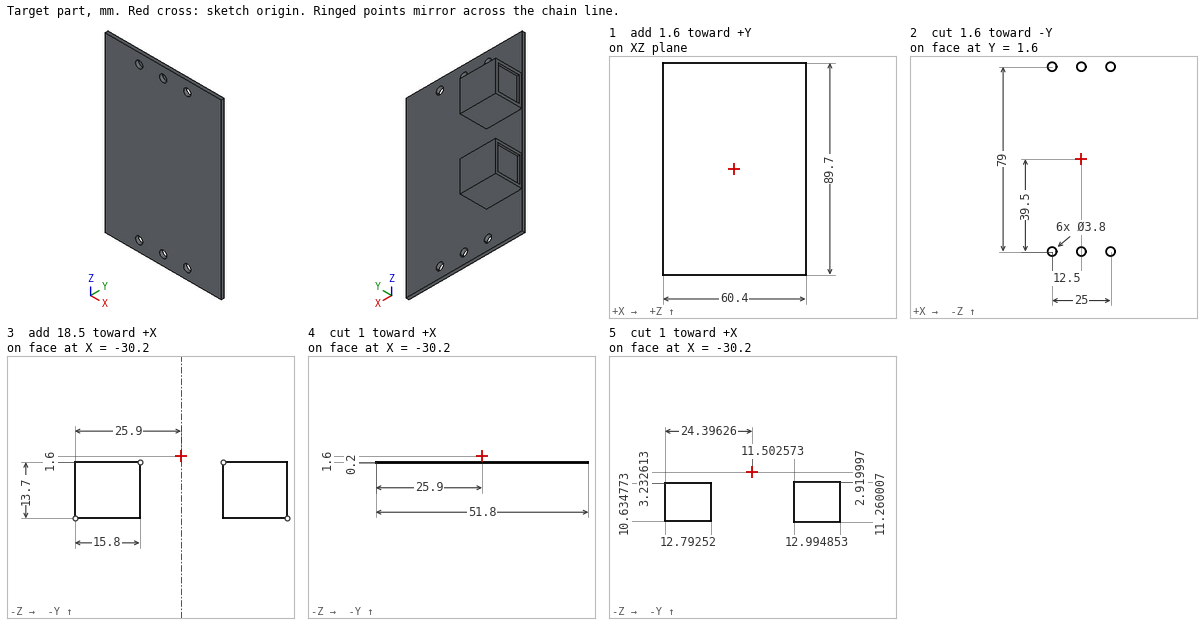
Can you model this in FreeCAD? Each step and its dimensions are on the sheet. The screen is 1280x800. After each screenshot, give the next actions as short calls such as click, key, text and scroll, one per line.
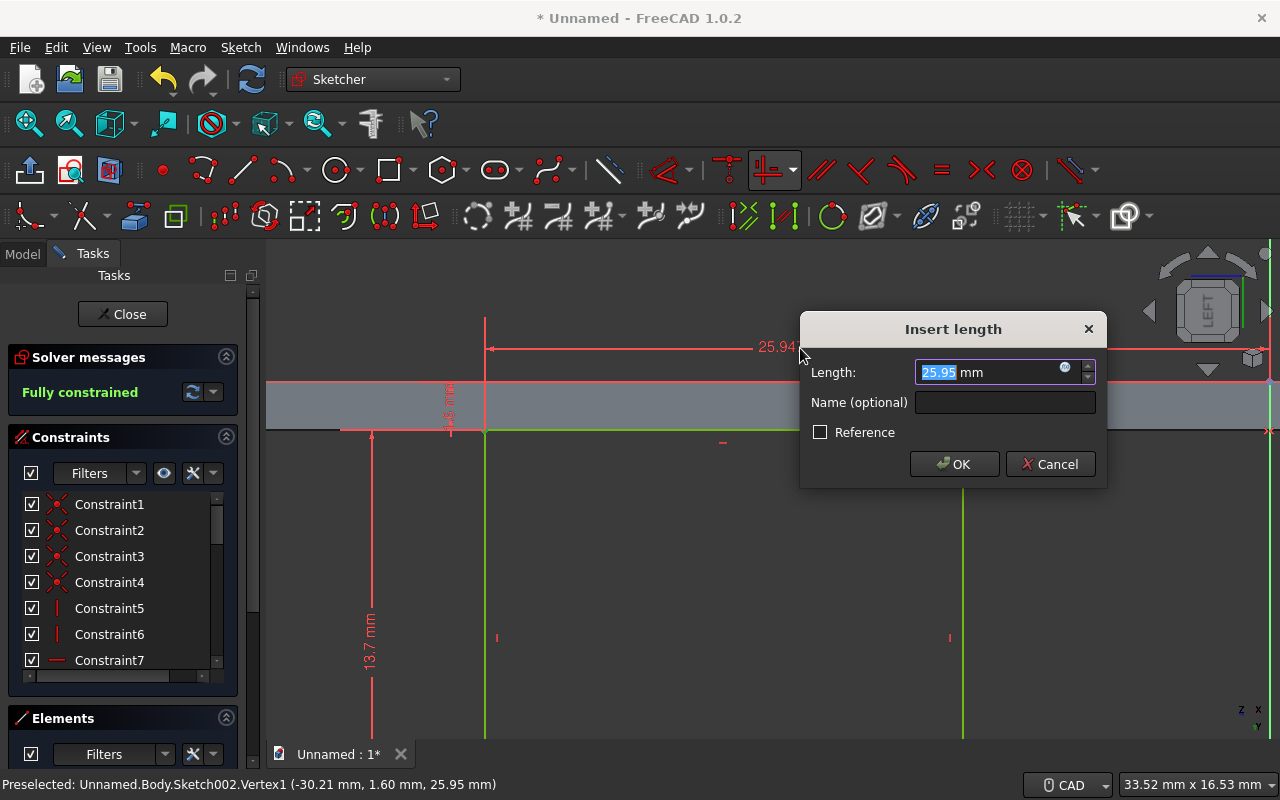
text(25.9)
key(Return)
key(Escape)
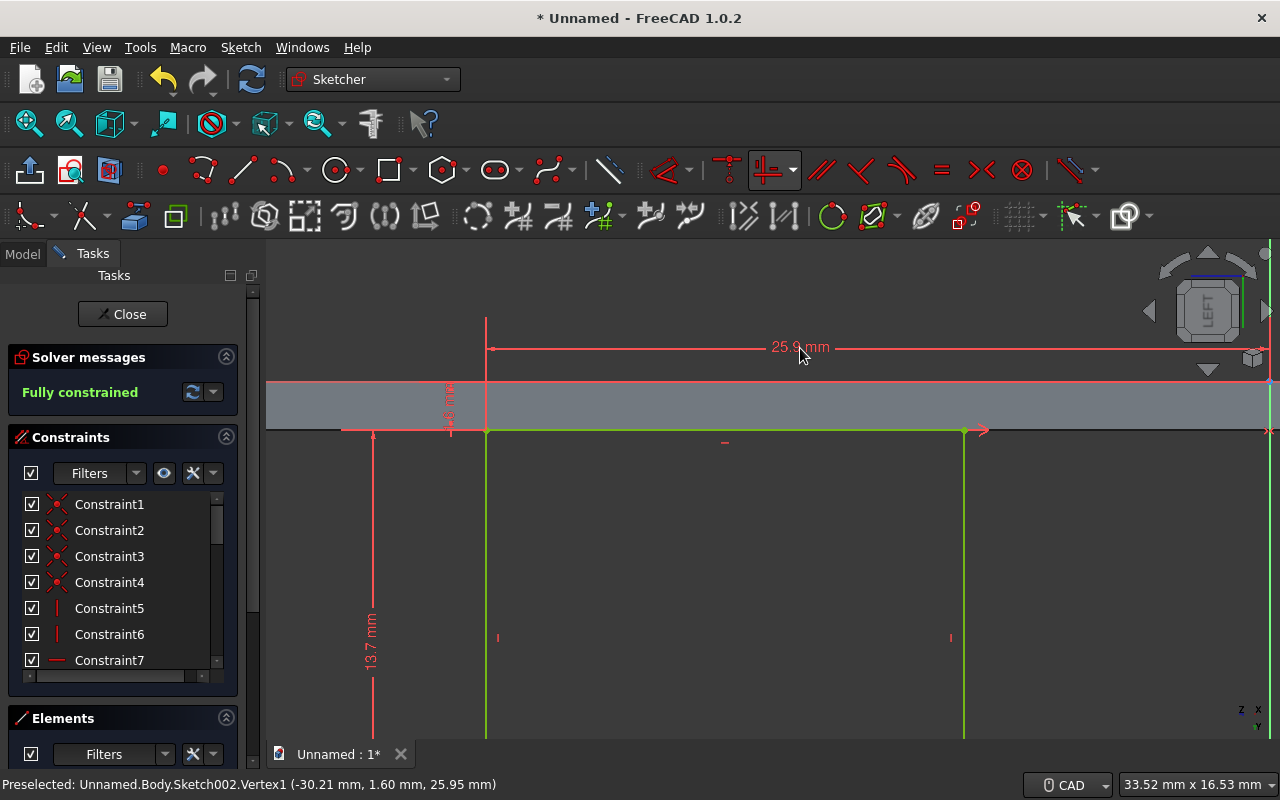
click(123, 314)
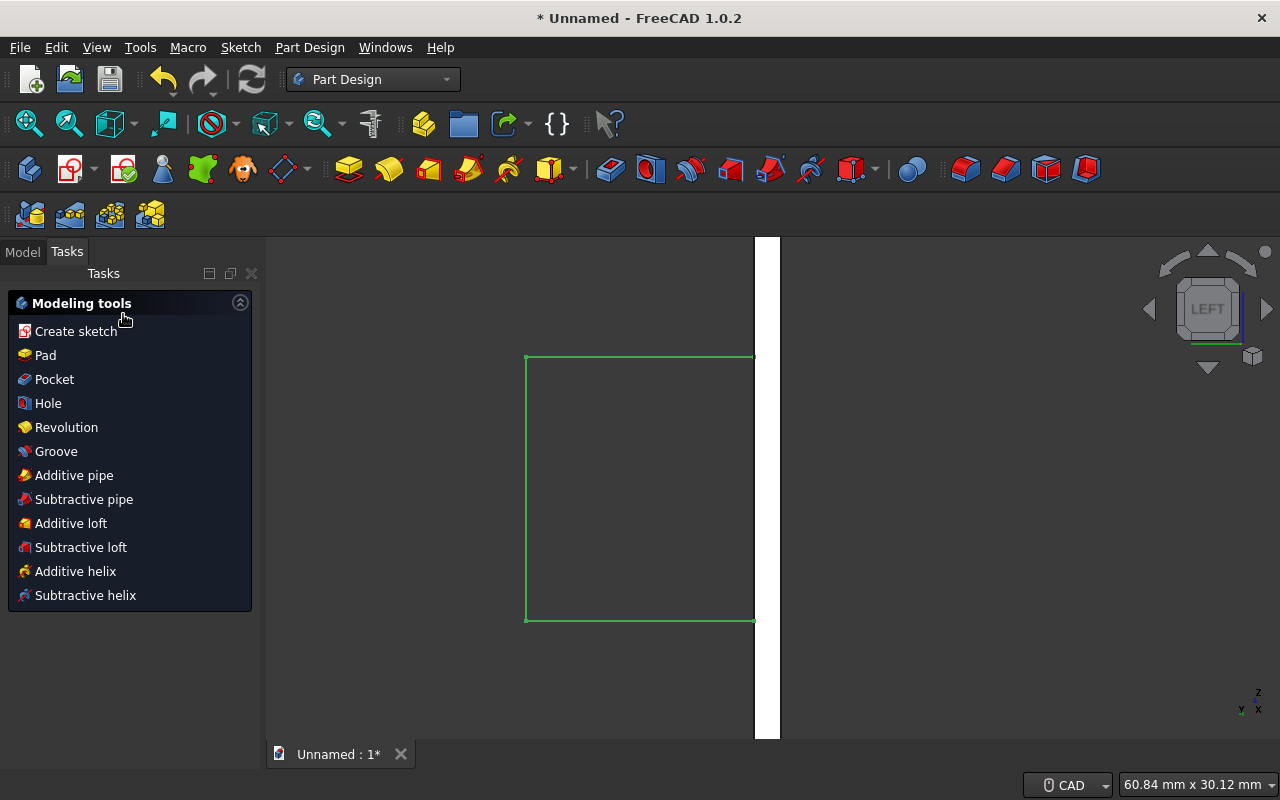
click(350, 170)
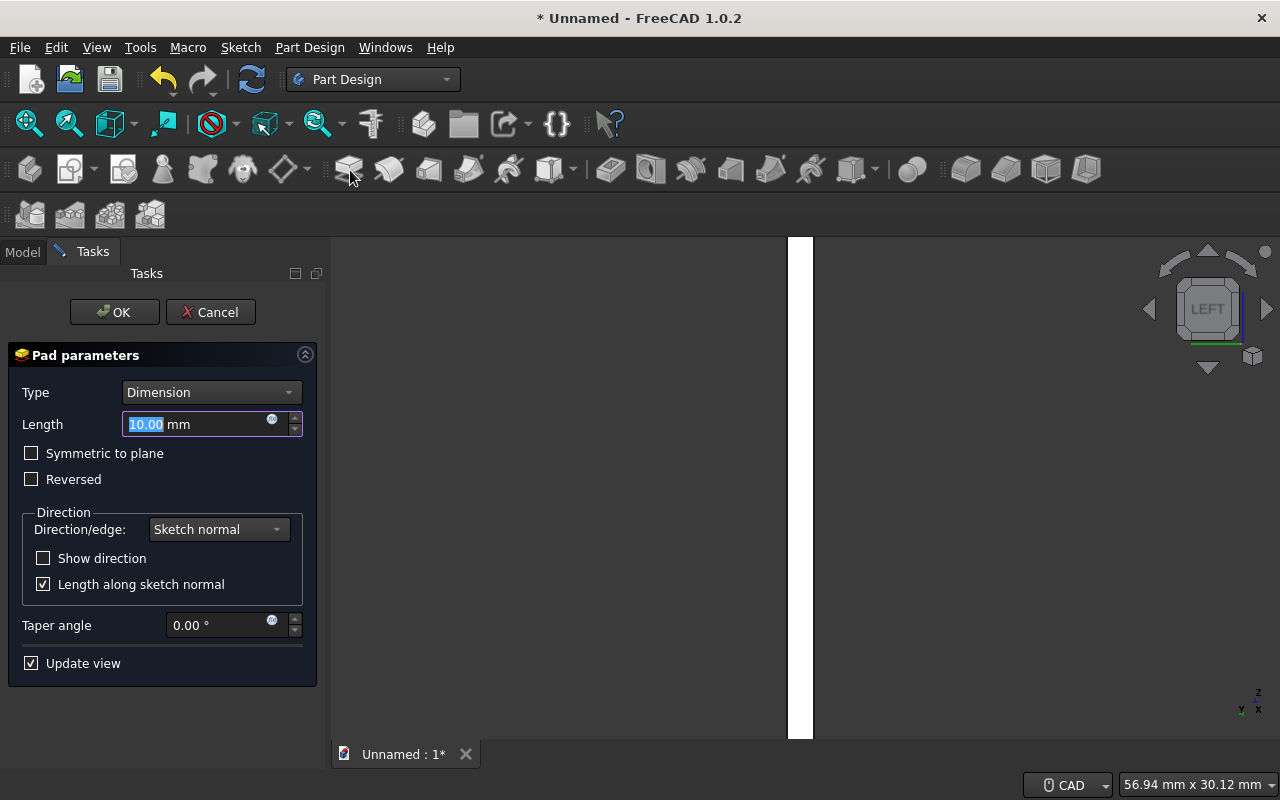
text(18.5)
key(Tab)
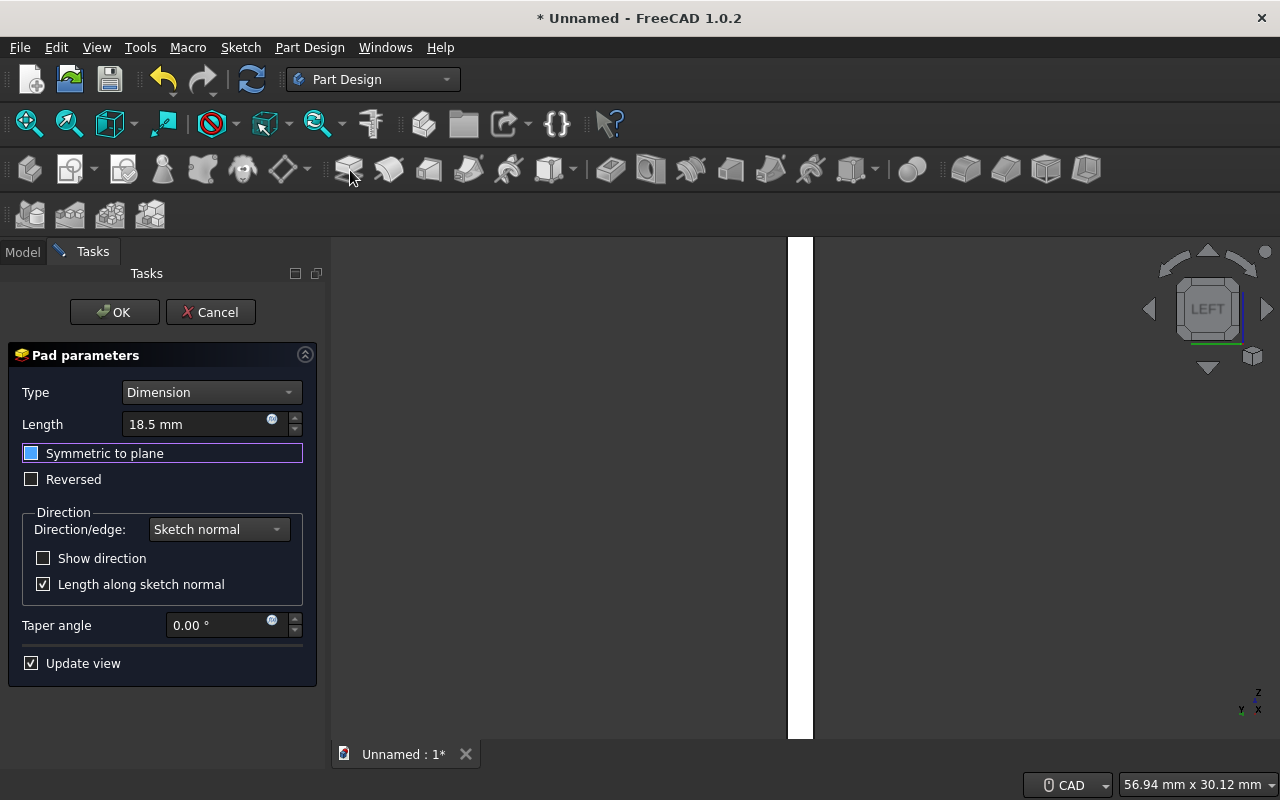
click(30, 479)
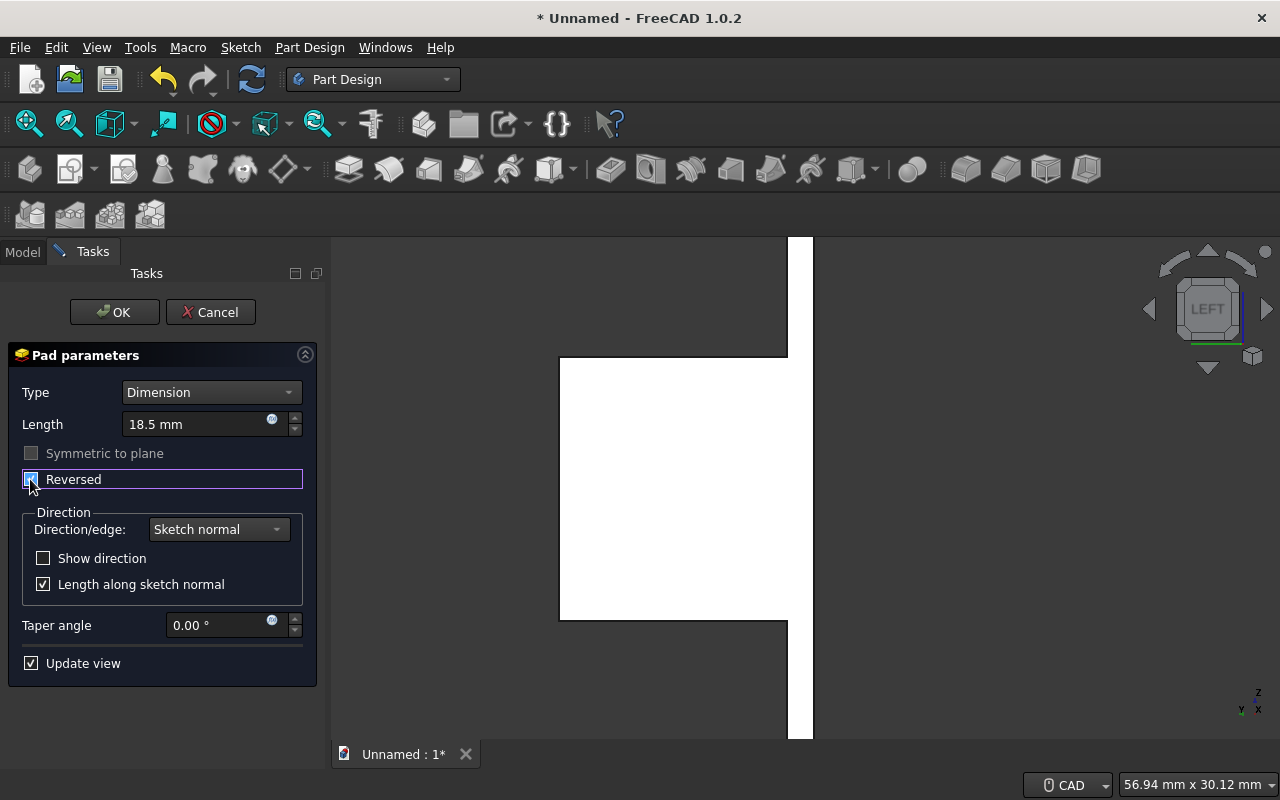
click(115, 312)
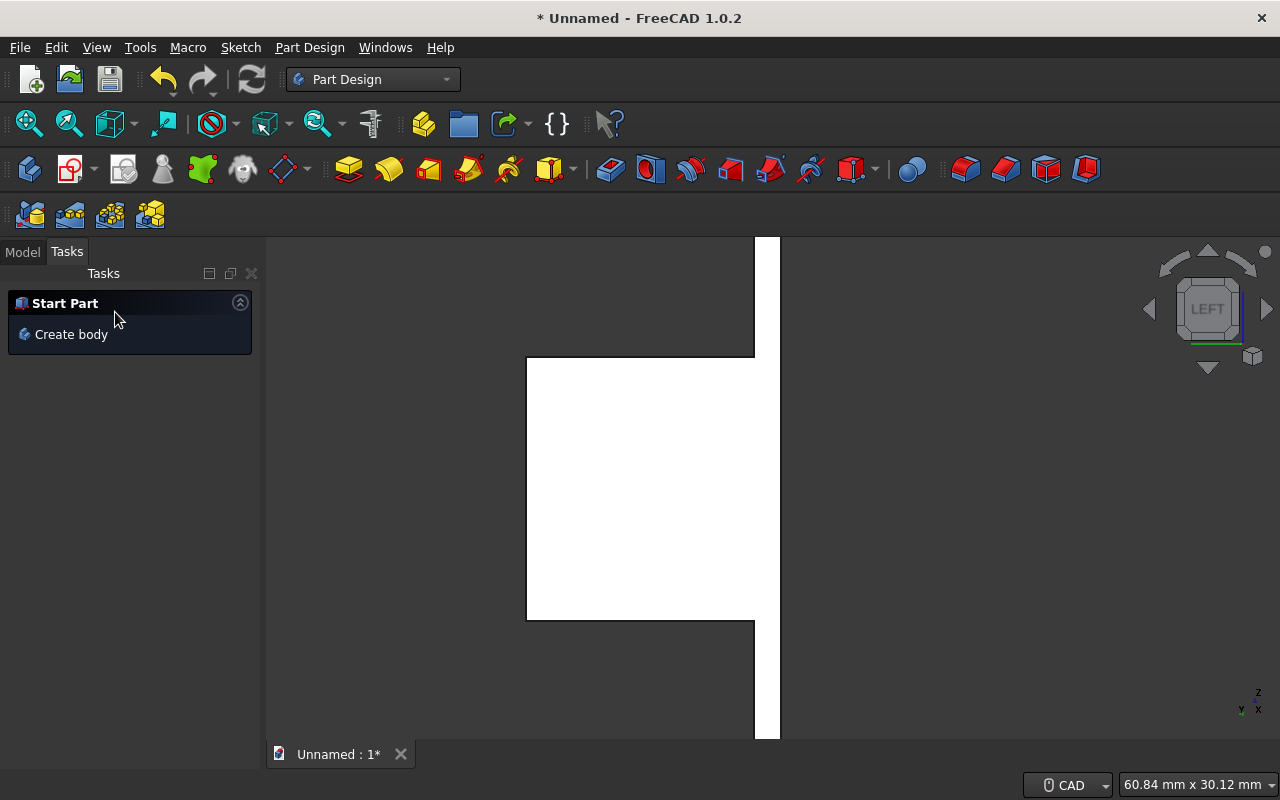
key(v)
key(f)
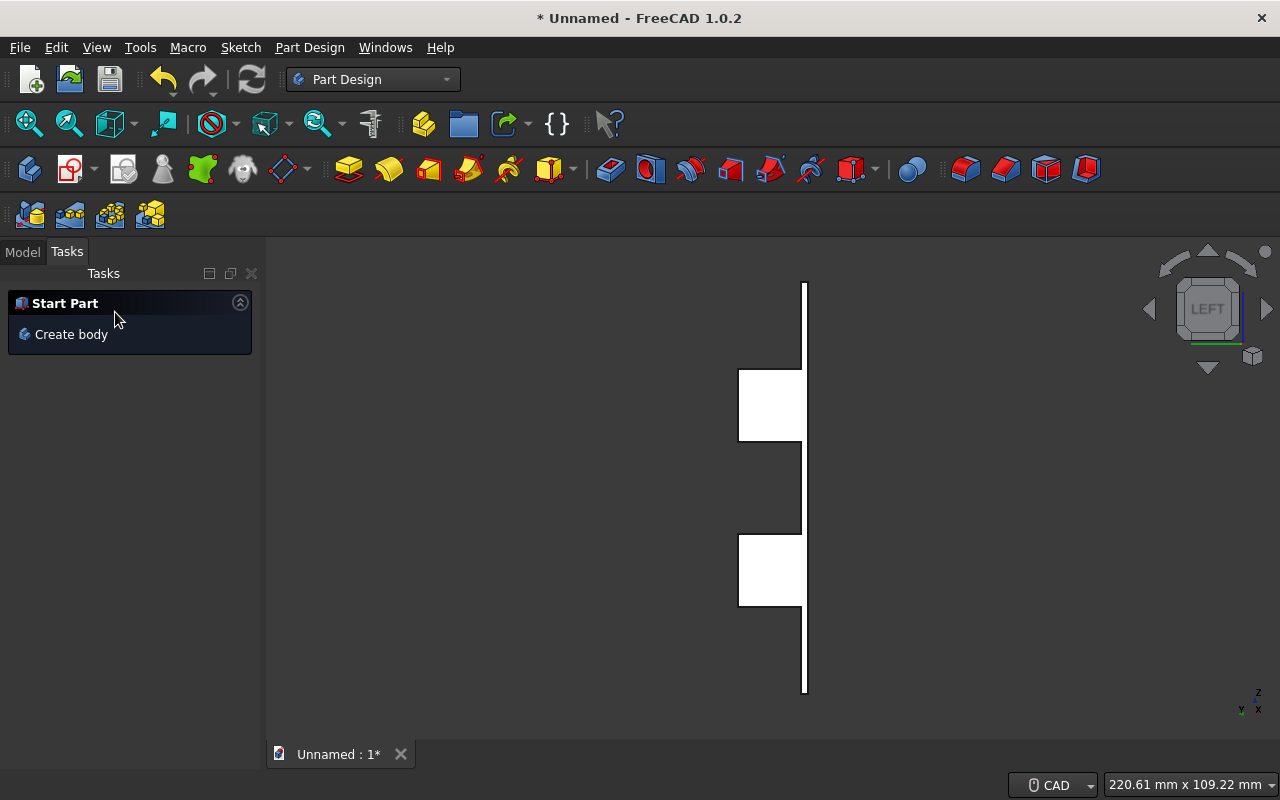
click(793, 546)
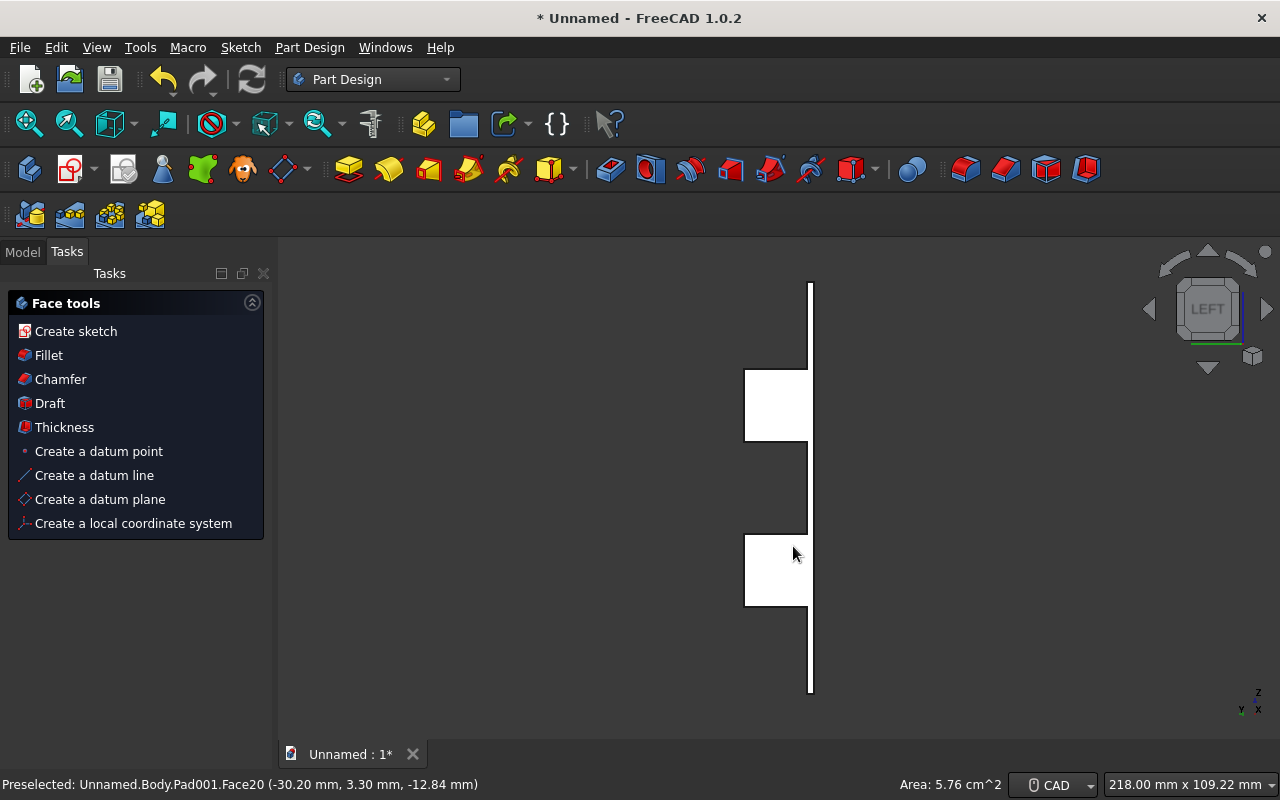
click(70, 170)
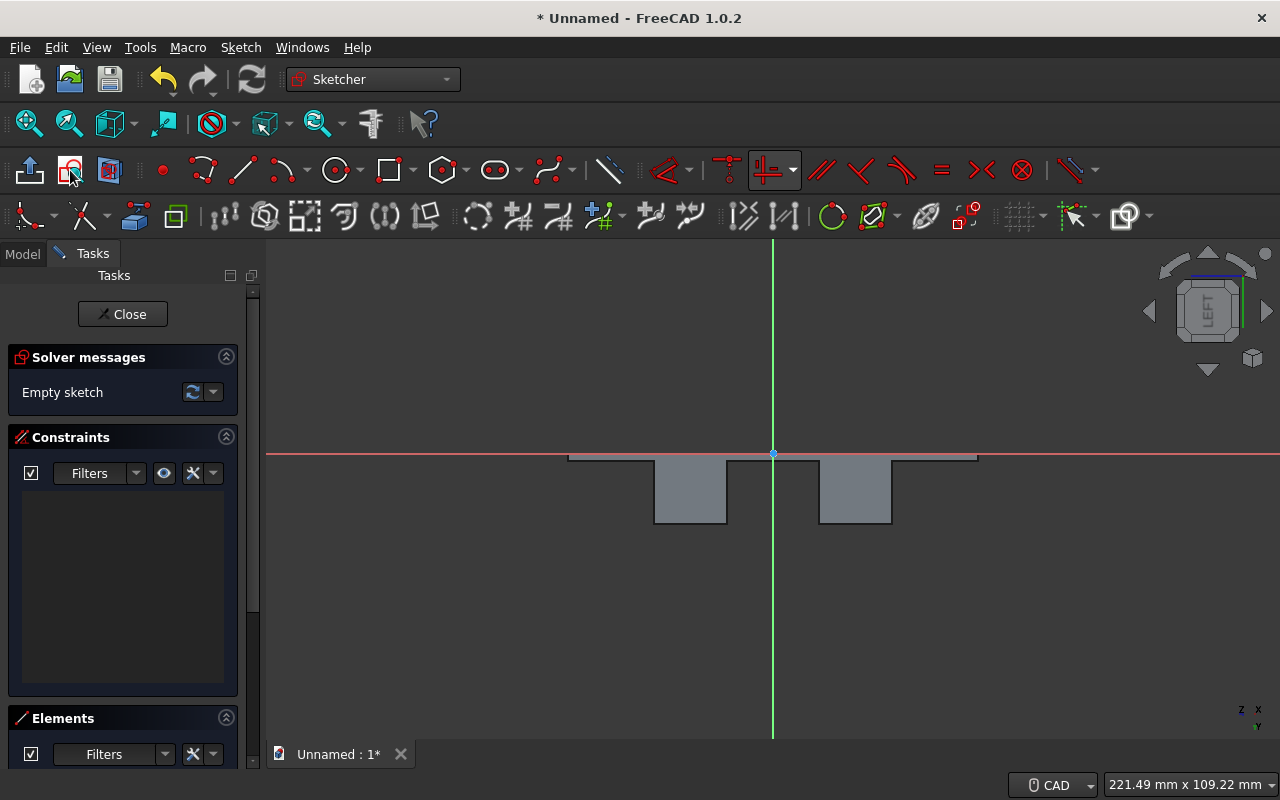
scroll(829, 433, up, 4)